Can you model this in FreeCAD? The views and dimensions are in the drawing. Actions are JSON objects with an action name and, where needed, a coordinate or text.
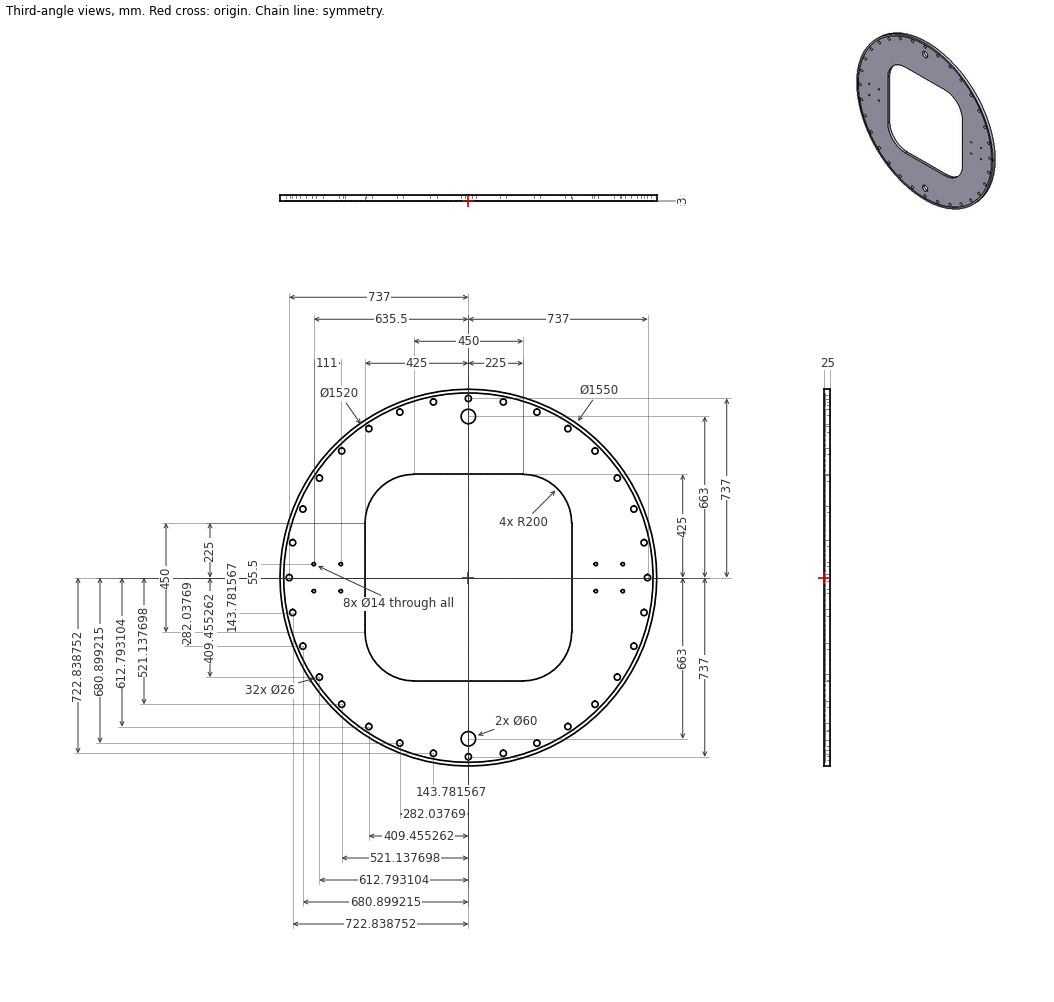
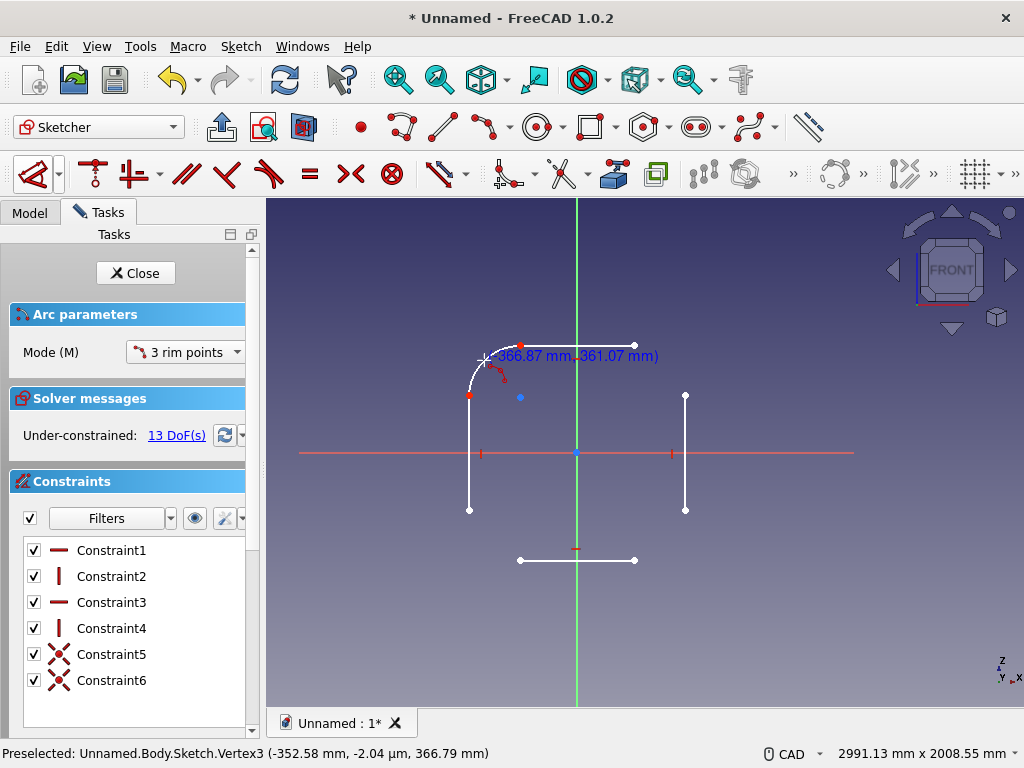
{"action": "left_click", "coordinate": [469, 511]}
{"action": "left_click", "coordinate": [520, 561]}
{"action": "left_click", "coordinate": [484, 545]}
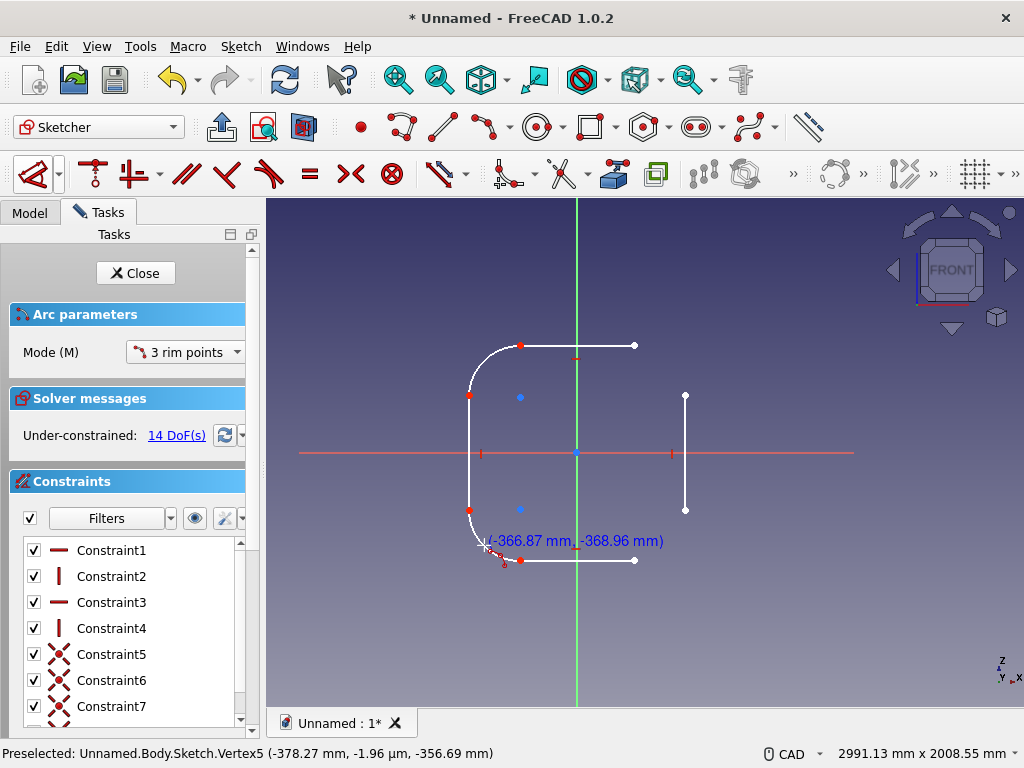
{"action": "left_click", "coordinate": [634, 561]}
{"action": "left_click", "coordinate": [685, 511]}
{"action": "left_click", "coordinate": [670, 545]}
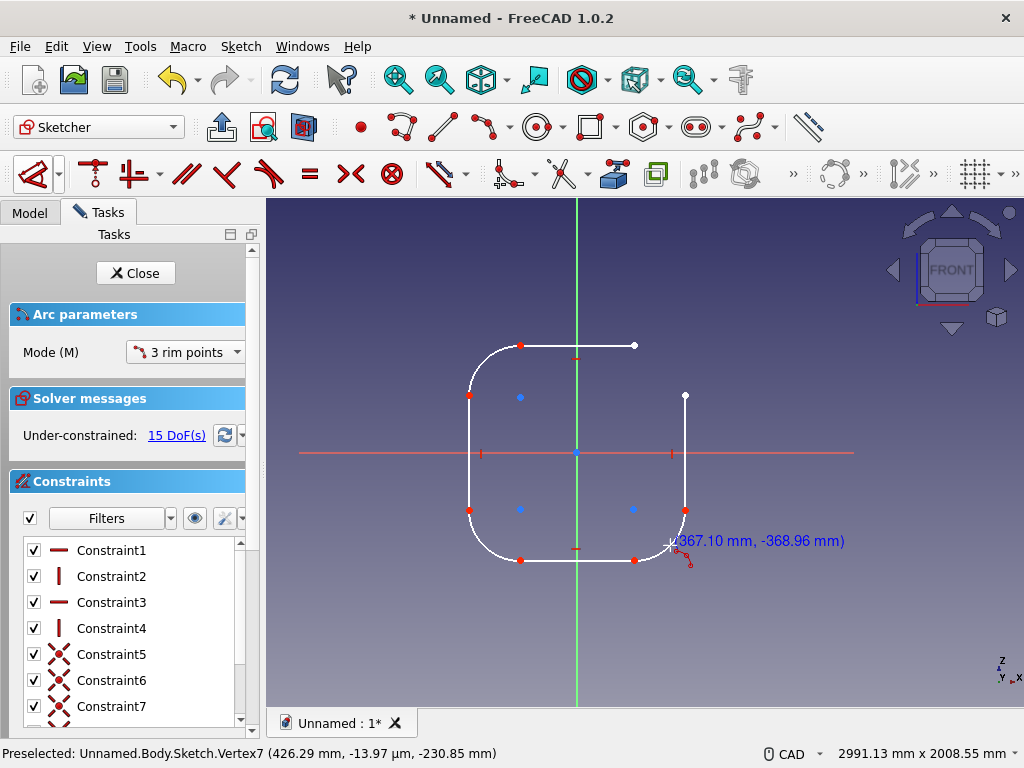
{"action": "left_click", "coordinate": [685, 396]}
{"action": "left_click", "coordinate": [634, 346]}
{"action": "left_click", "coordinate": [670, 360]}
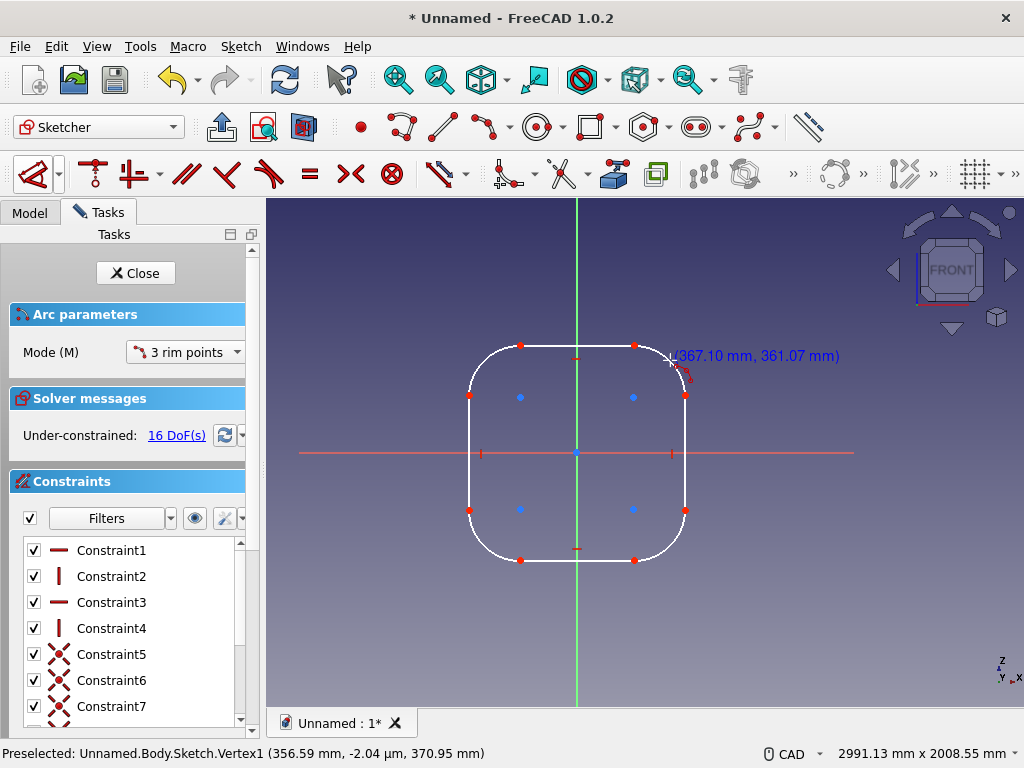
{"action": "left_click", "coordinate": [536, 128]}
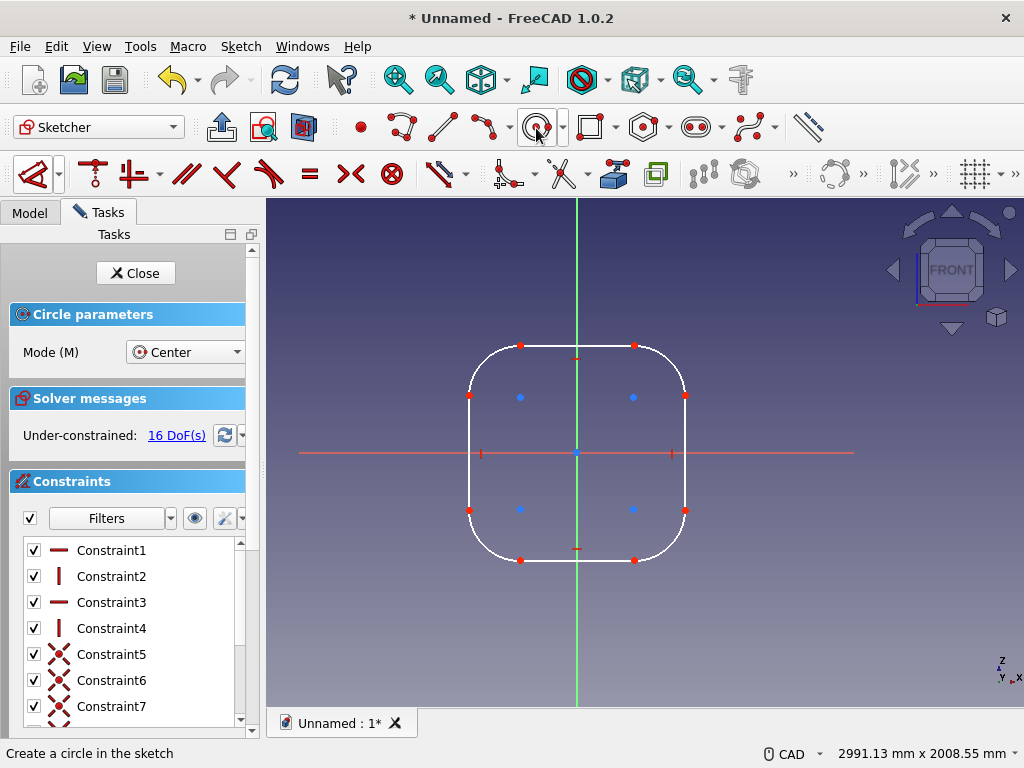
{"action": "left_click", "coordinate": [577, 452]}
{"action": "left_click", "coordinate": [716, 314]}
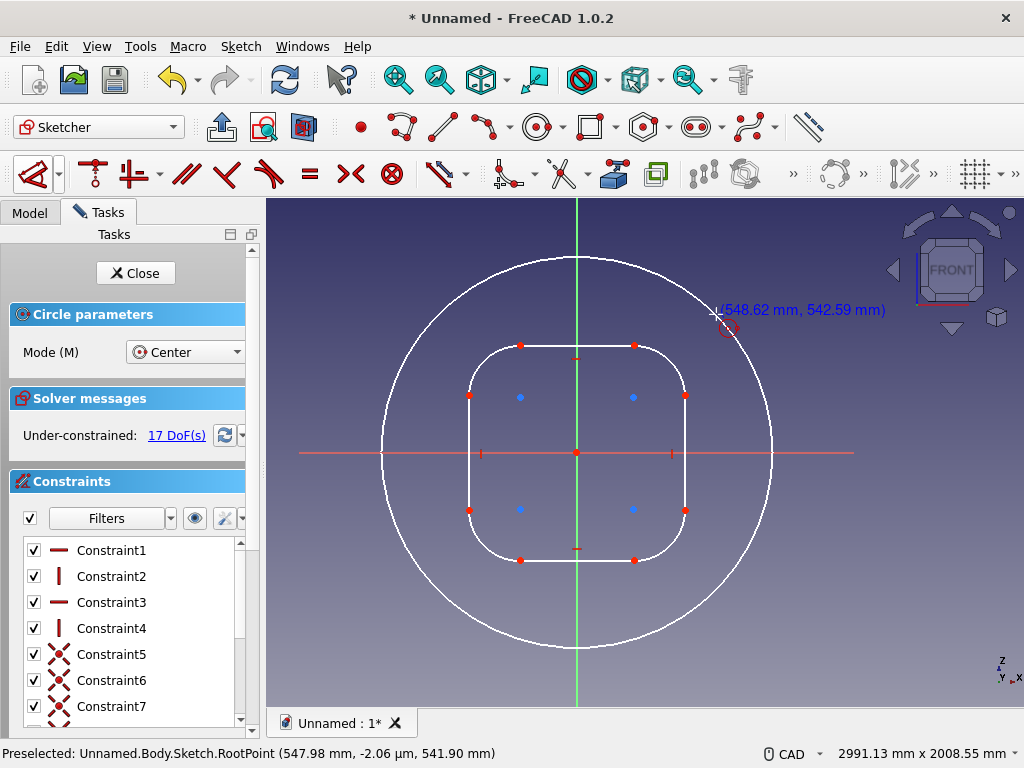
{"action": "scroll", "coordinate": [422, 556], "scroll_direction": "up", "scroll_amount": 10}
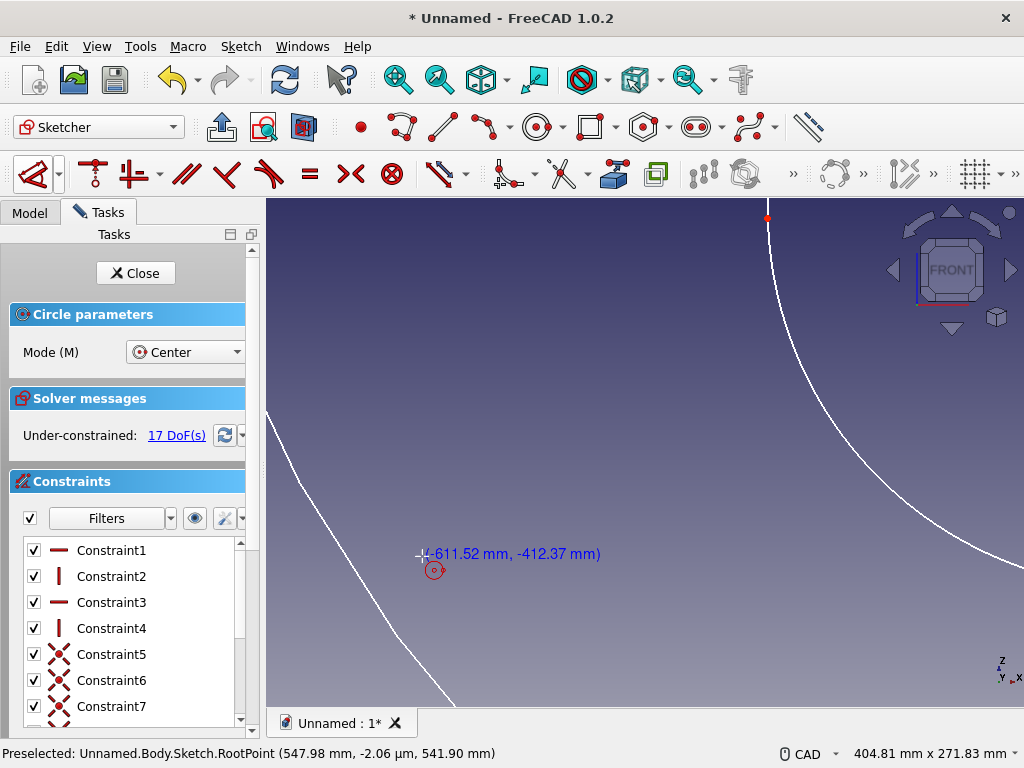
{"action": "scroll", "coordinate": [453, 535], "scroll_direction": "down", "scroll_amount": 11}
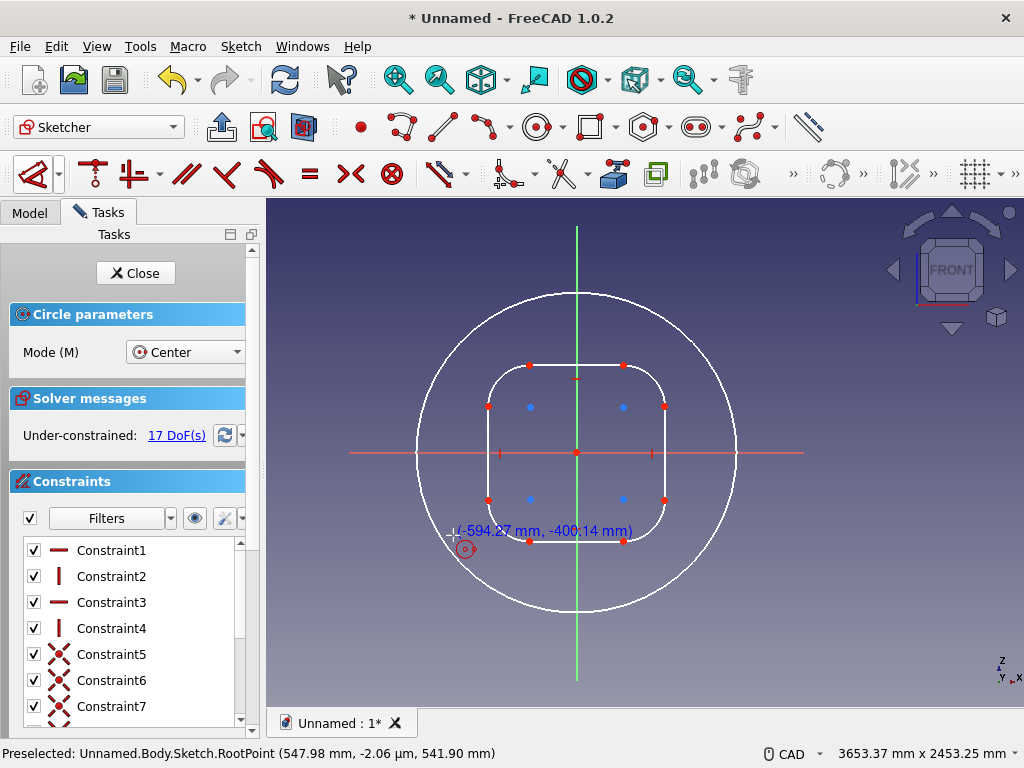
{"action": "scroll", "coordinate": [449, 538], "scroll_direction": "up", "scroll_amount": 4}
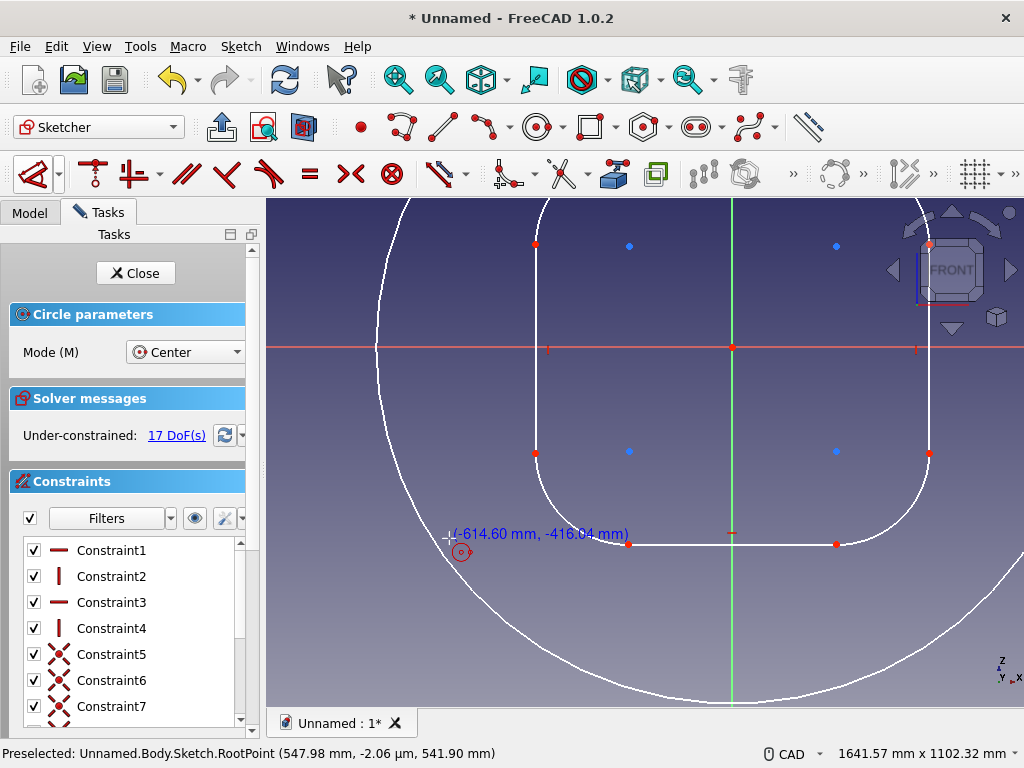
{"action": "left_click", "coordinate": [450, 536]}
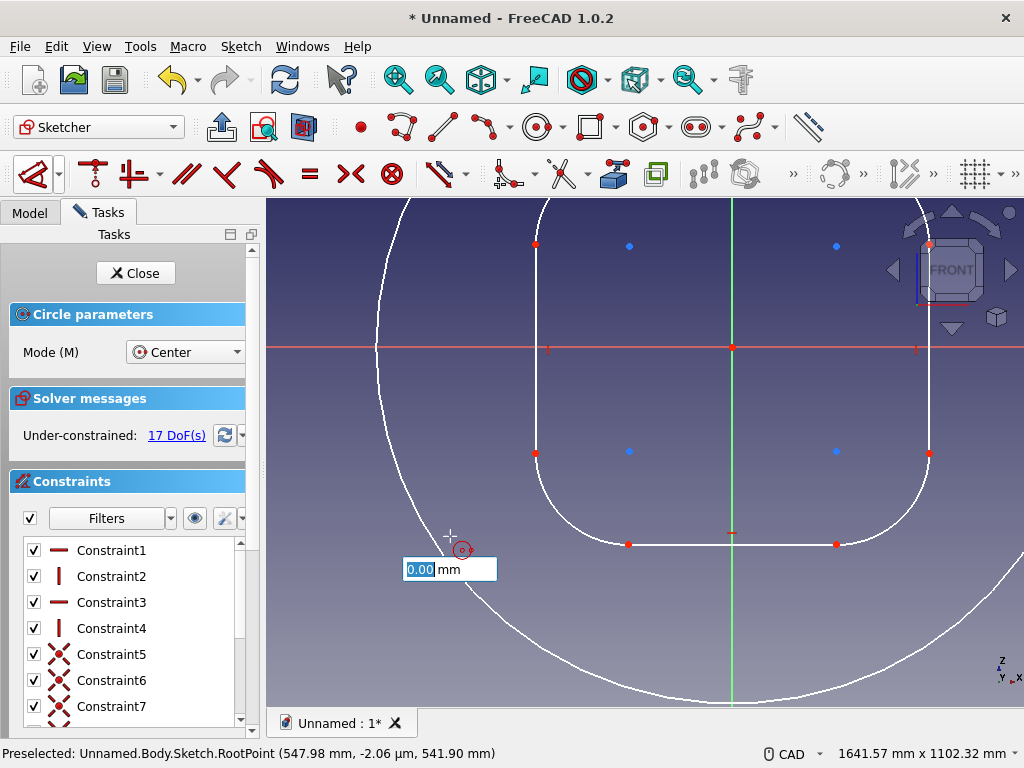
{"action": "scroll", "coordinate": [454, 532], "scroll_direction": "up", "scroll_amount": 5}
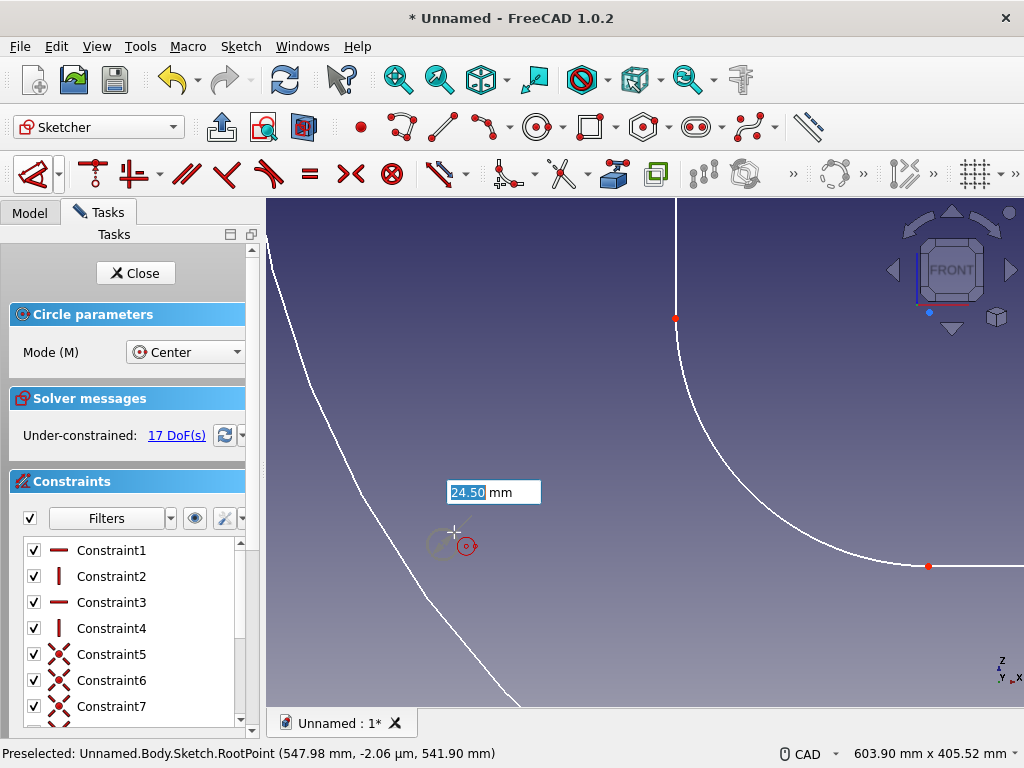
{"action": "left_click", "coordinate": [453, 531]}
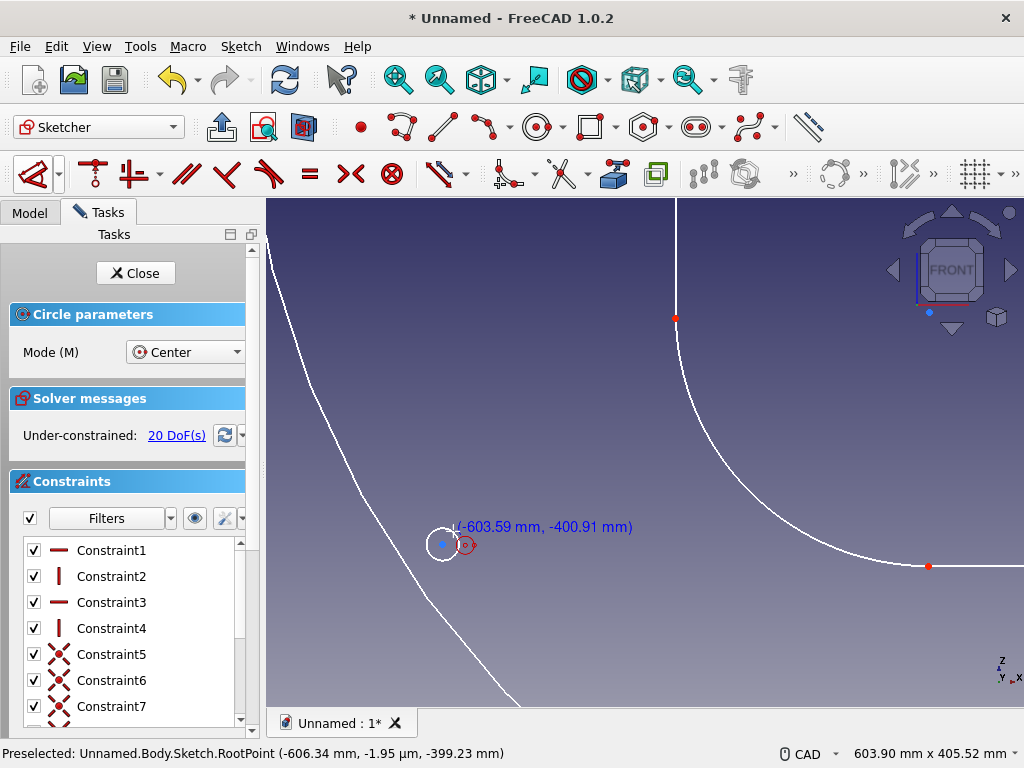
{"action": "scroll", "coordinate": [451, 536], "scroll_direction": "down", "scroll_amount": 9}